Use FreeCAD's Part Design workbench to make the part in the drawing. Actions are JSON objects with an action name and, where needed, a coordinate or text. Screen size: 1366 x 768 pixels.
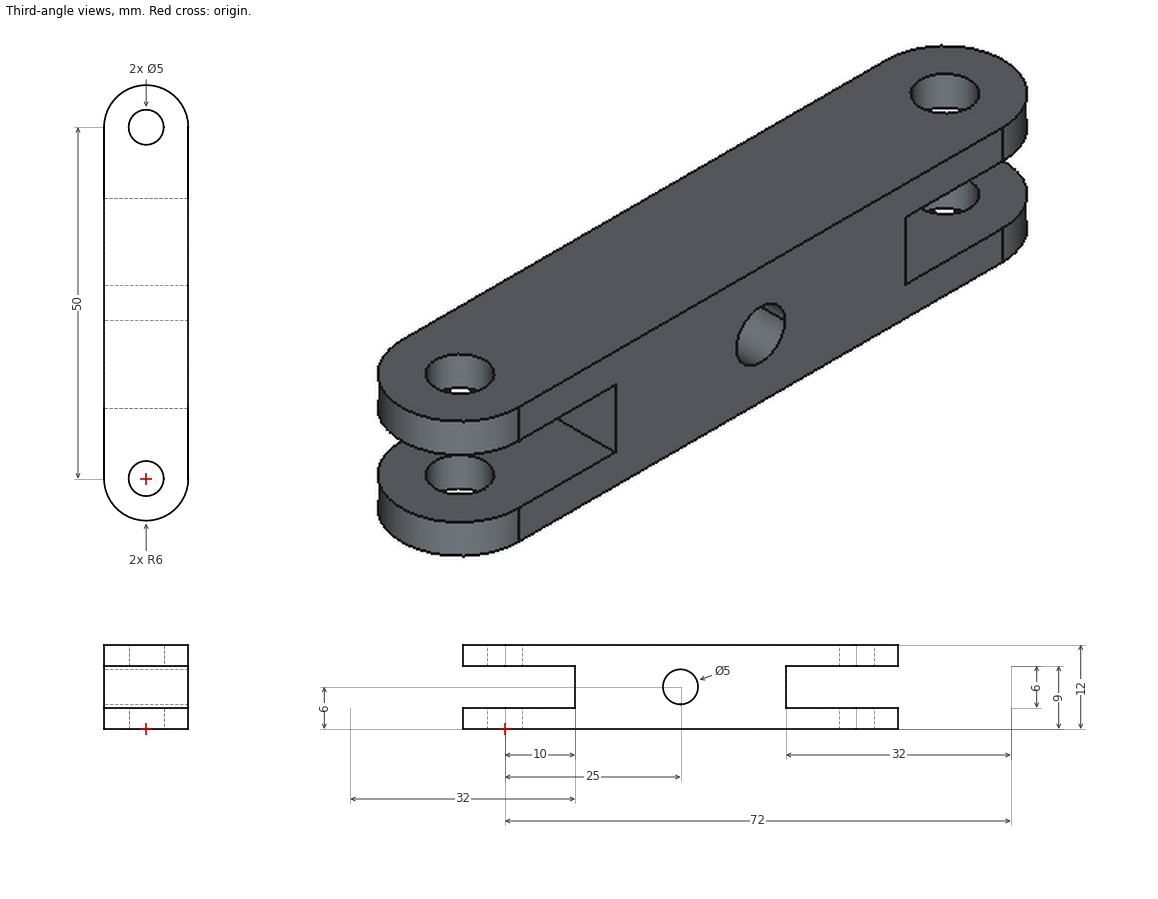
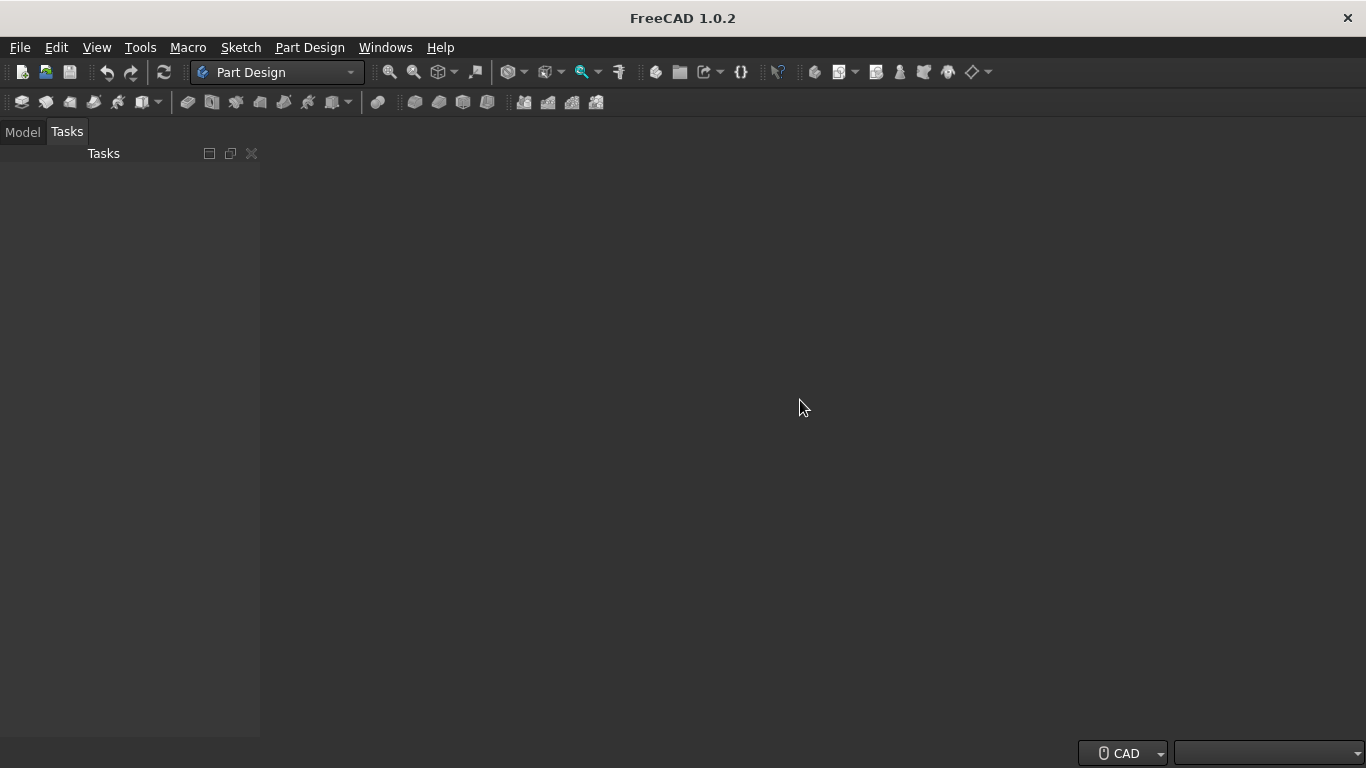
{"action": "key", "text": "ctrl+n"}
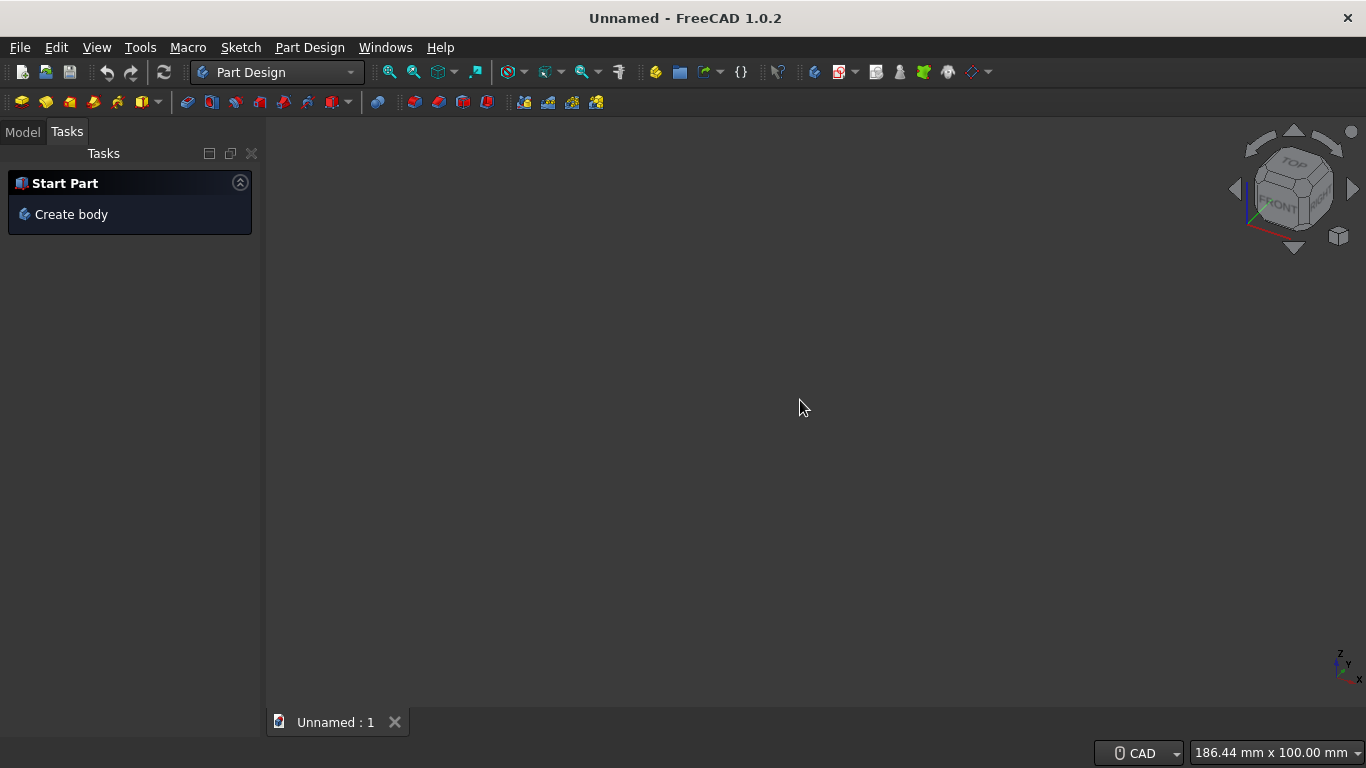
{"action": "left_click", "coordinate": [840, 72]}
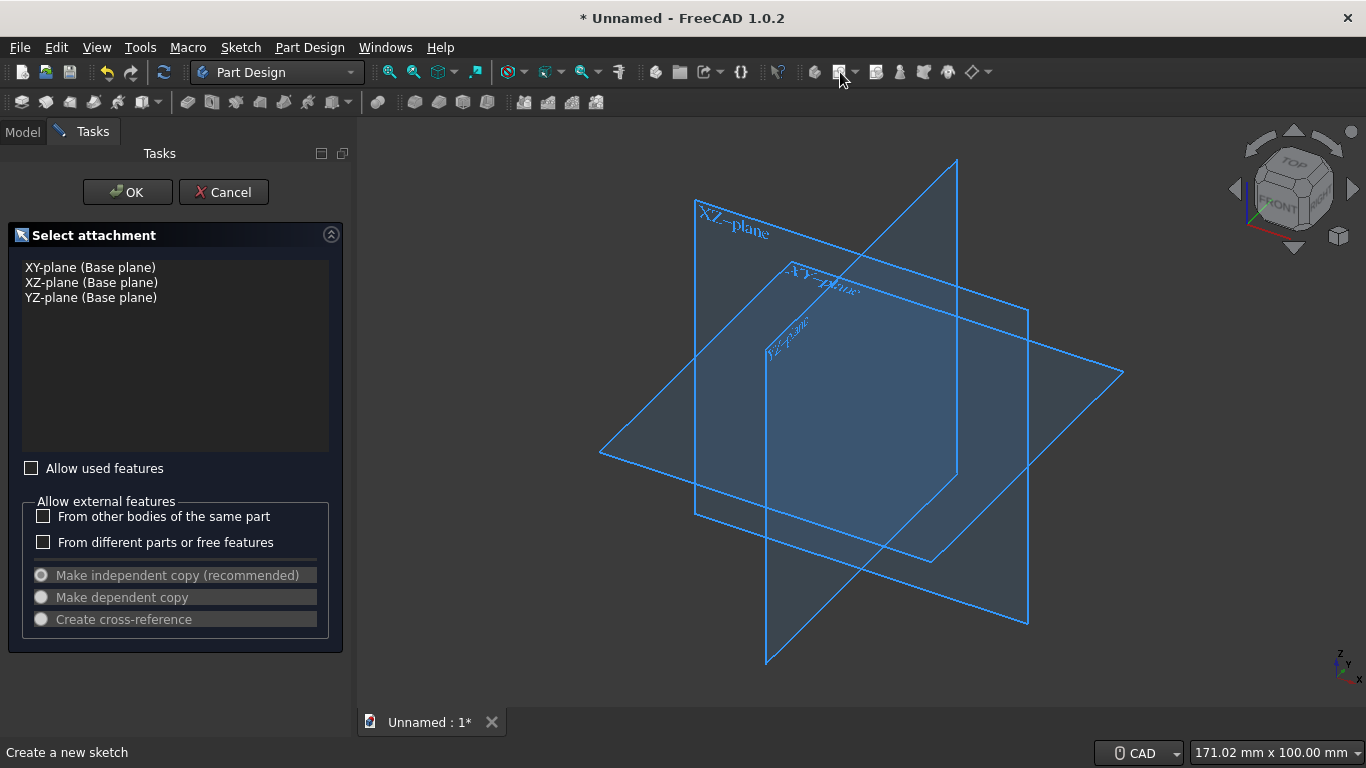
{"action": "left_click", "coordinate": [82, 268]}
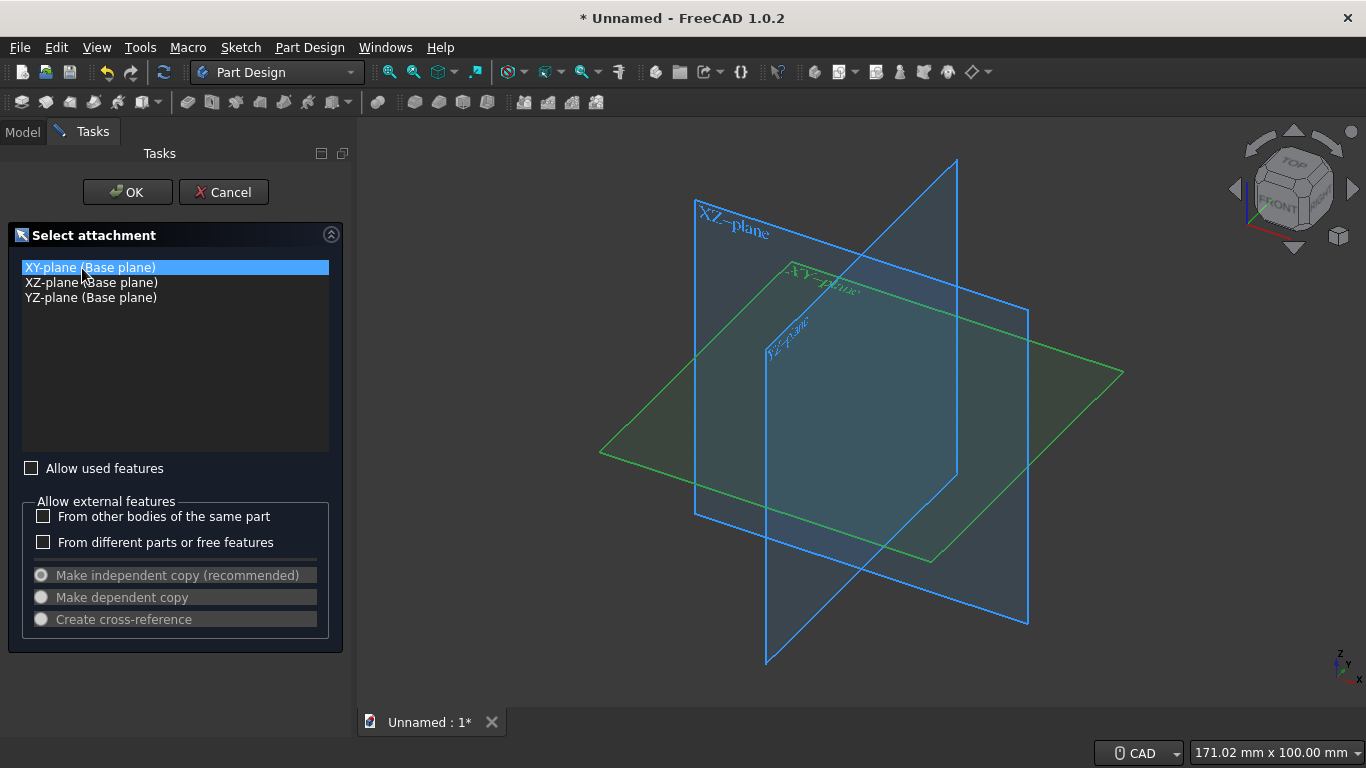
{"action": "left_click", "coordinate": [128, 192]}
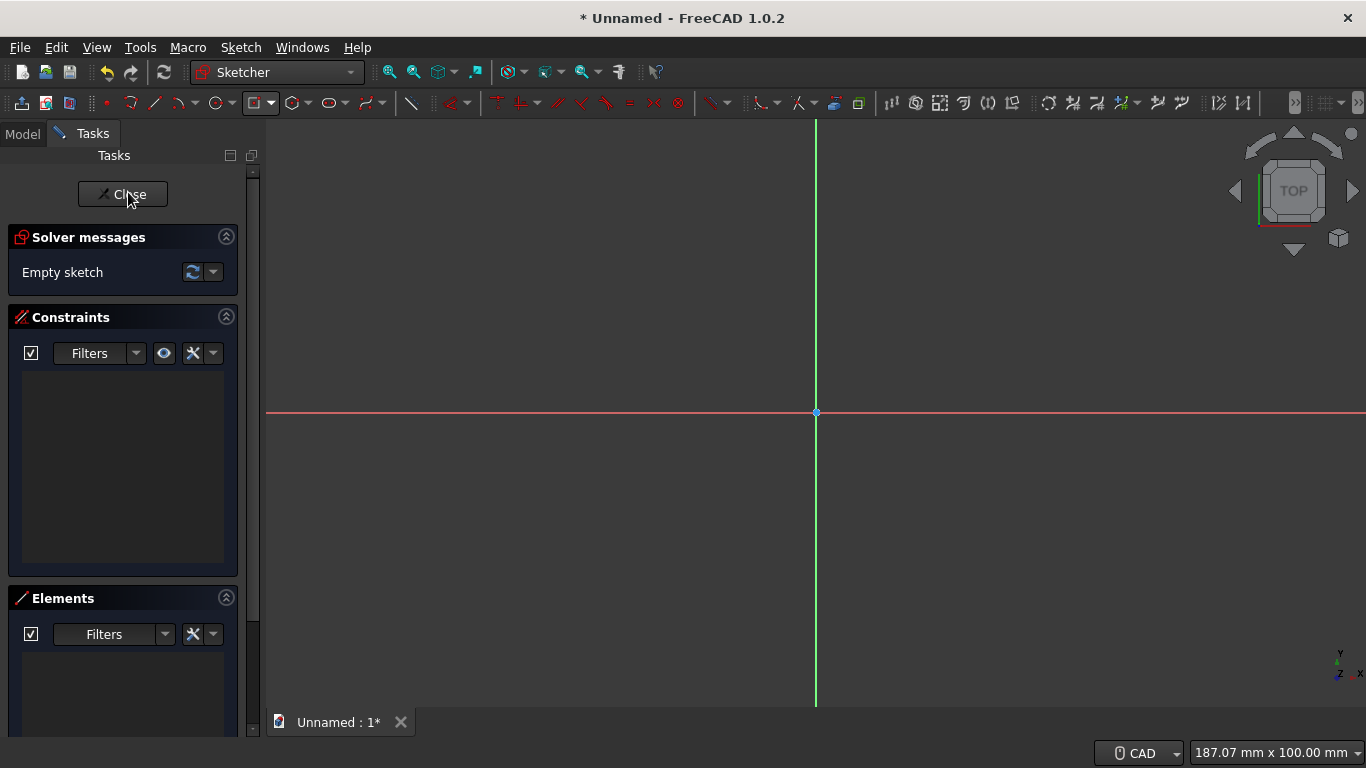
{"action": "scroll", "coordinate": [438, 679], "scroll_direction": "down", "scroll_amount": 1}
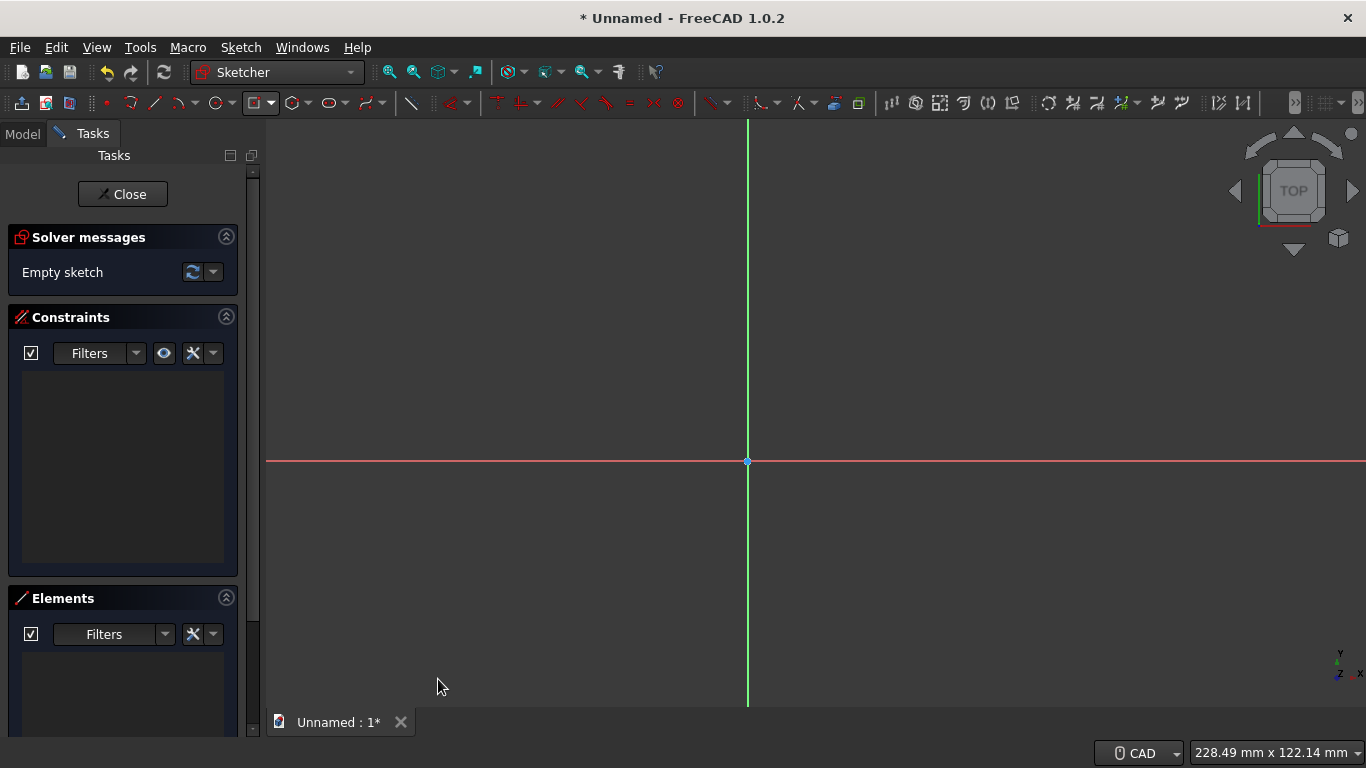
{"action": "key", "text": "g s"}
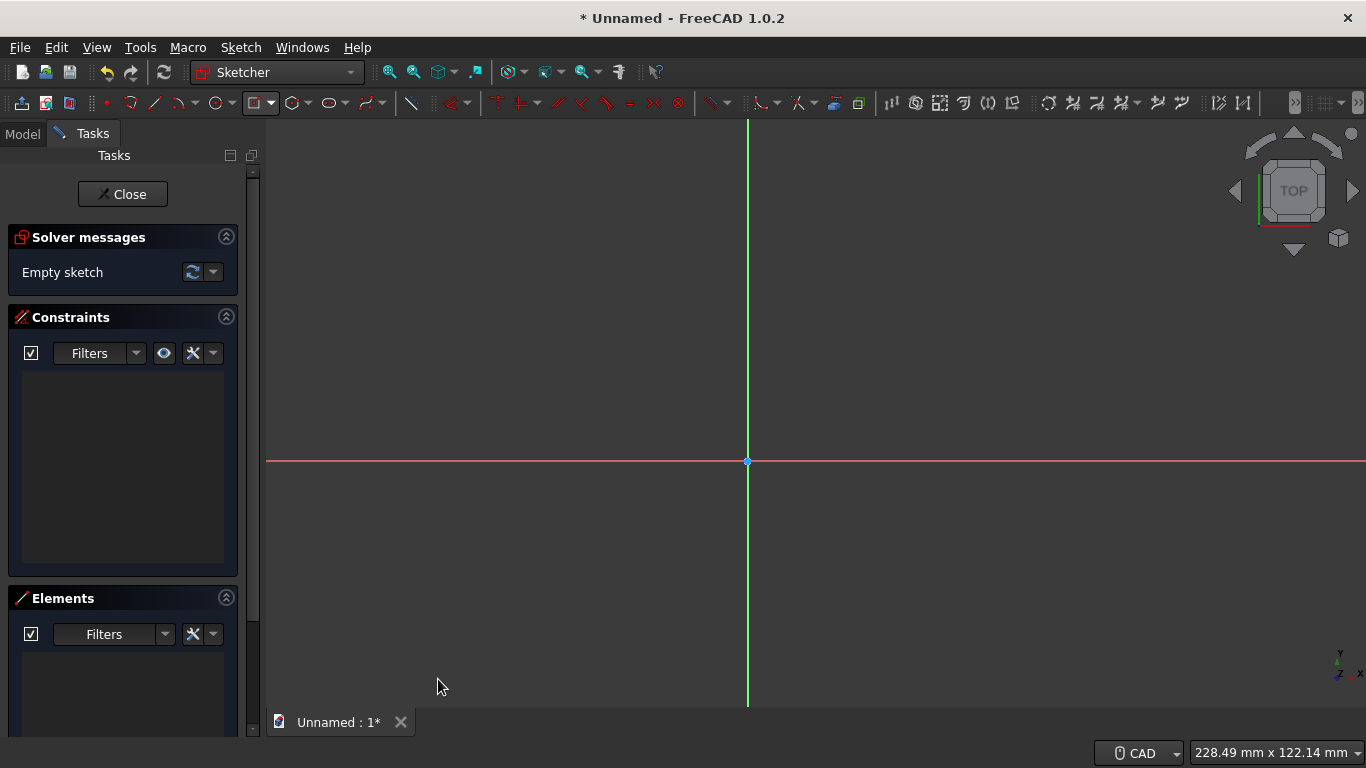
{"action": "left_click", "coordinate": [748, 461]}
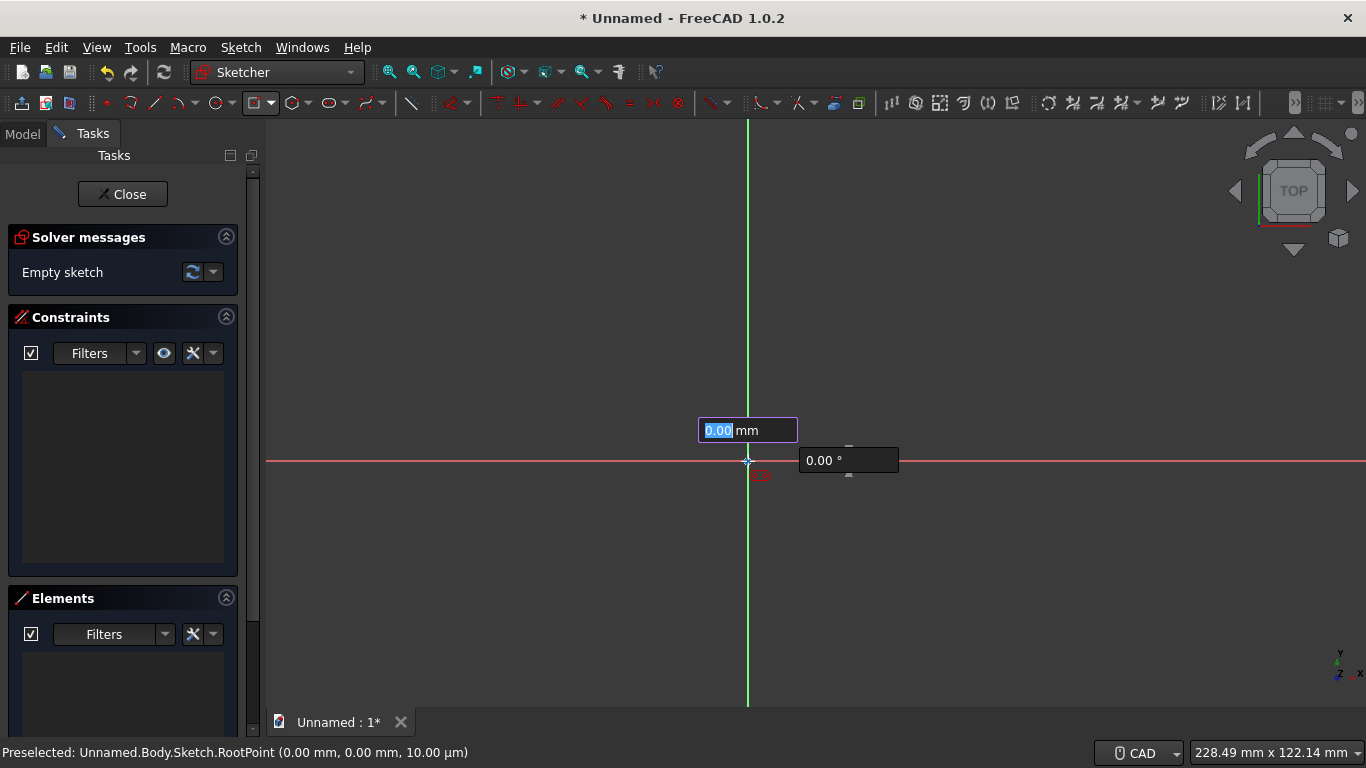
{"action": "left_click", "coordinate": [757, 221]}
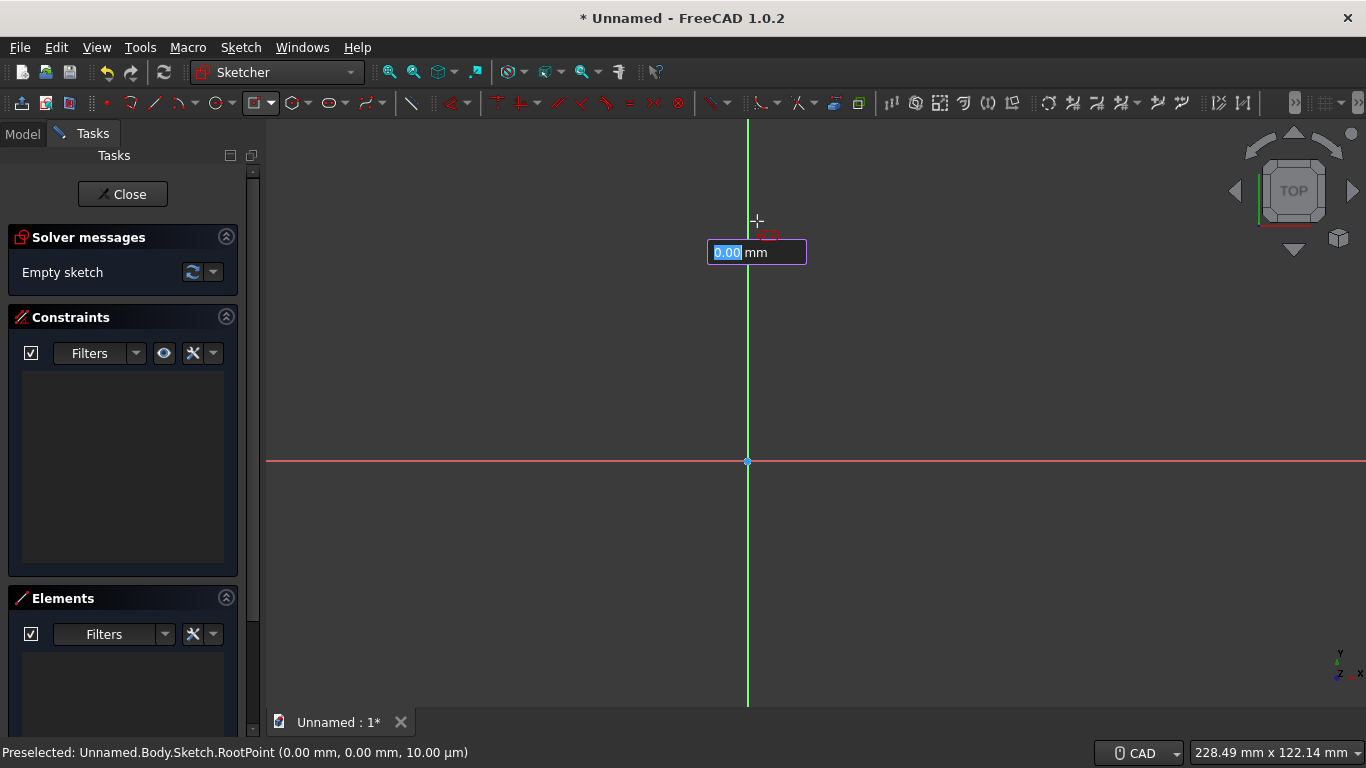
{"action": "left_click", "coordinate": [719, 341]}
{"action": "key", "text": "Escape"}